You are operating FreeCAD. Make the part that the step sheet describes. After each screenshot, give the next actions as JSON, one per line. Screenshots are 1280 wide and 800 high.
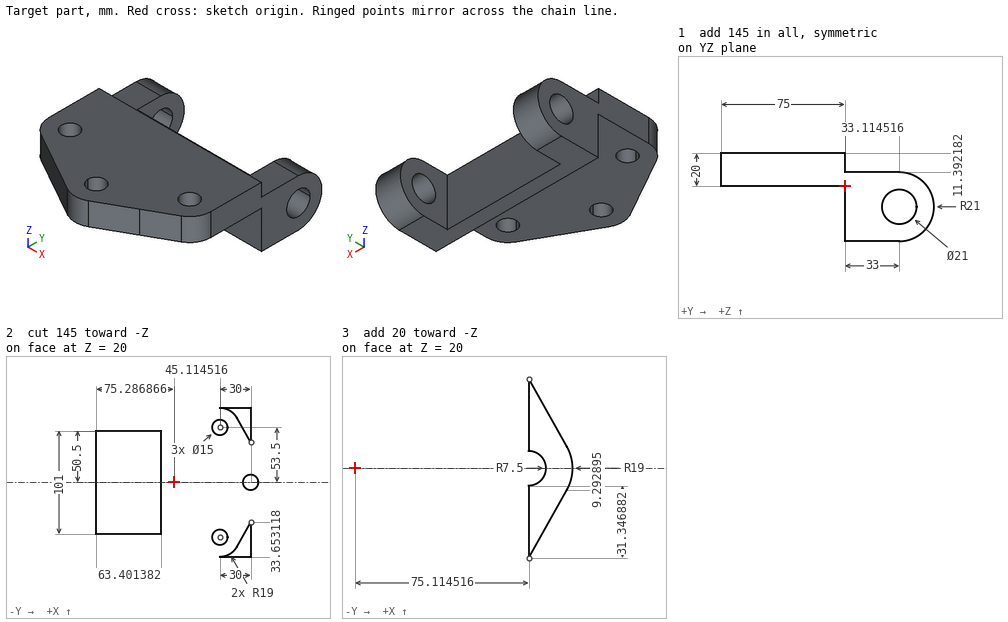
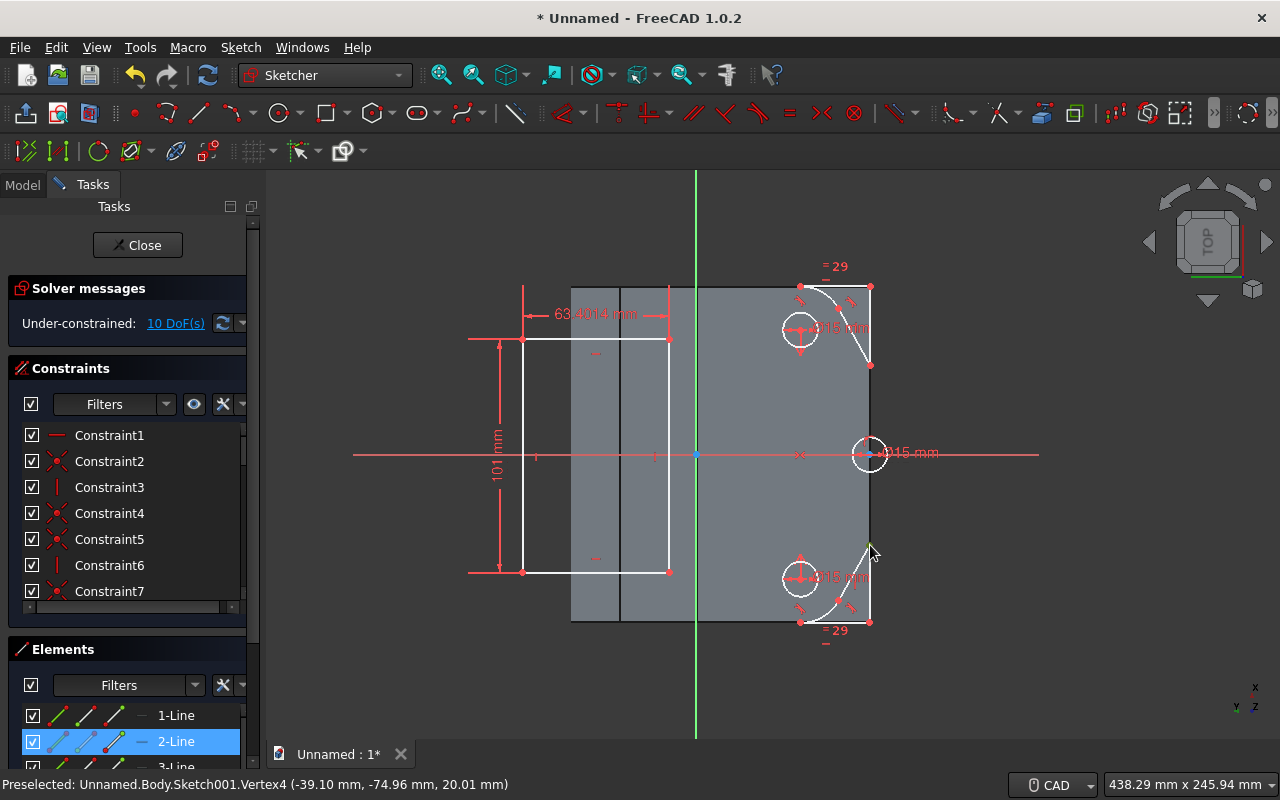
{"action": "left_click", "coordinate": [870, 366]}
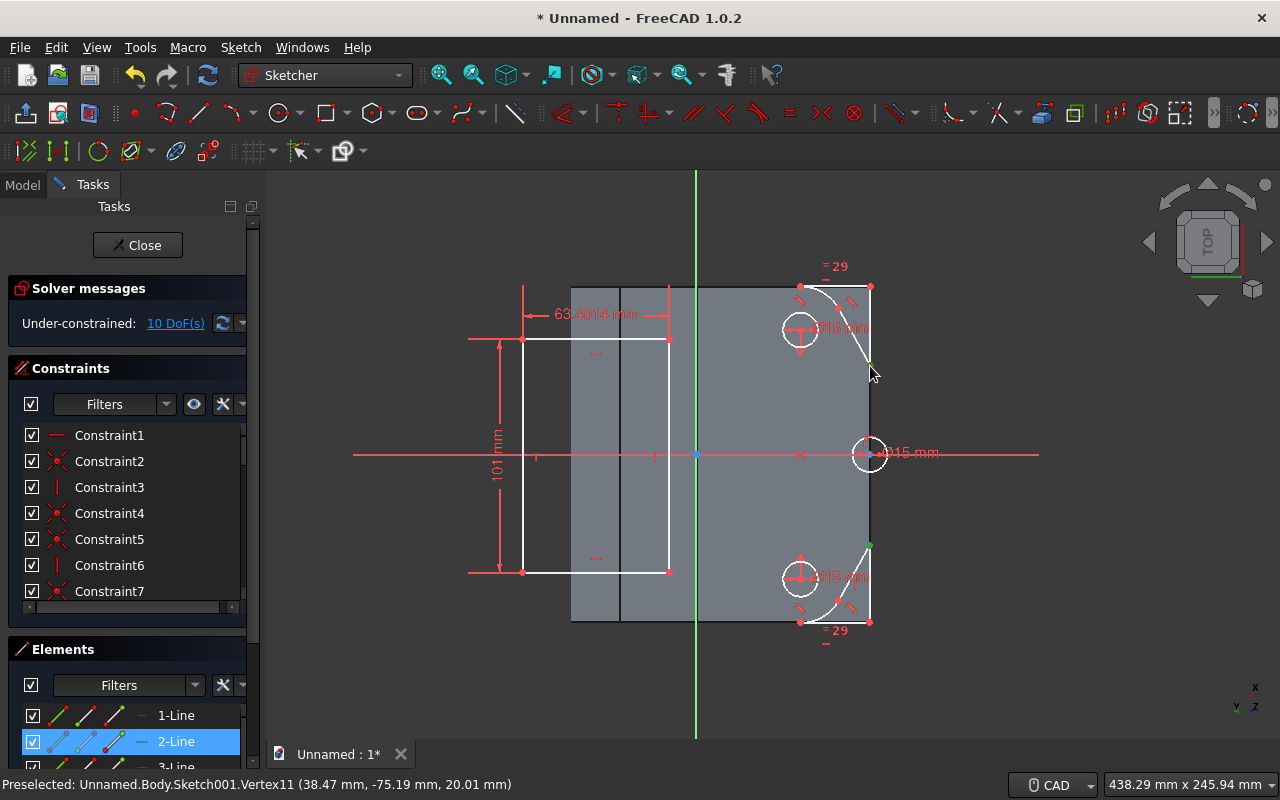
{"action": "left_click", "coordinate": [353, 455]}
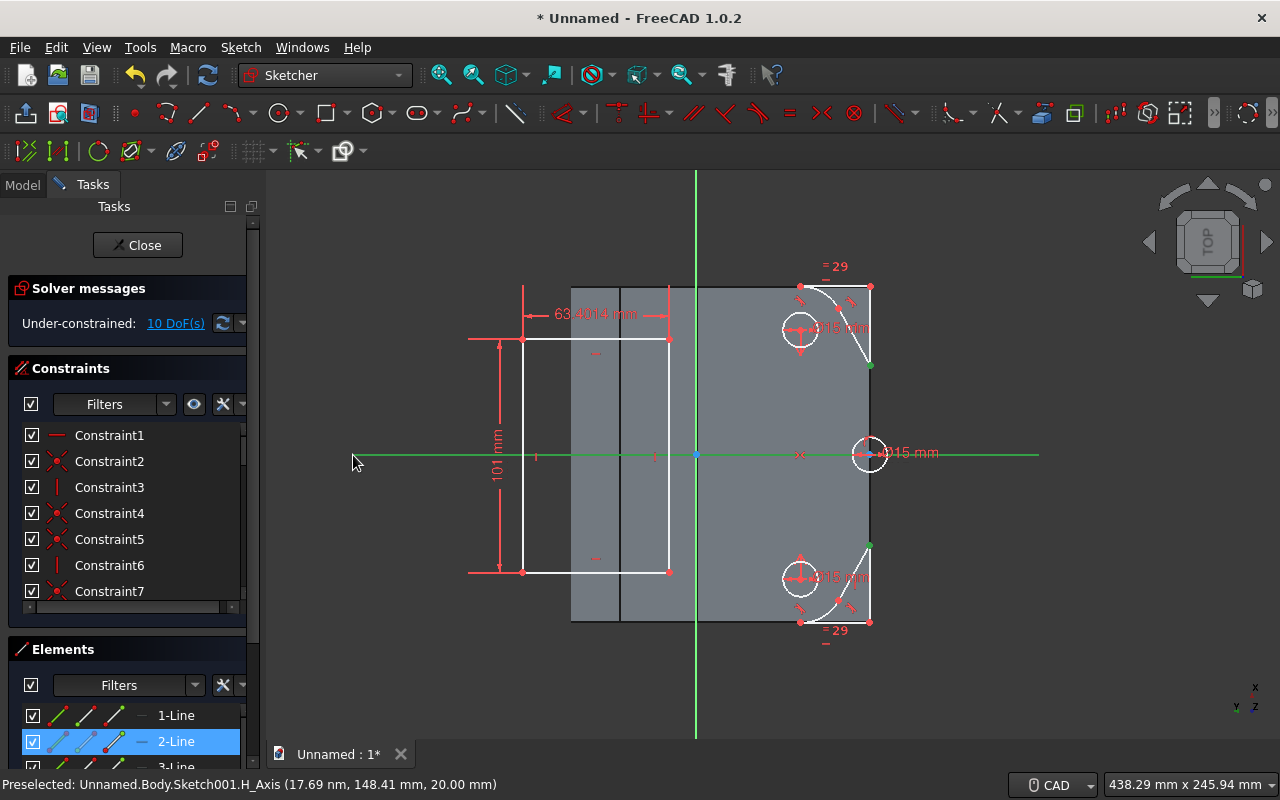
{"action": "left_click", "coordinate": [822, 114]}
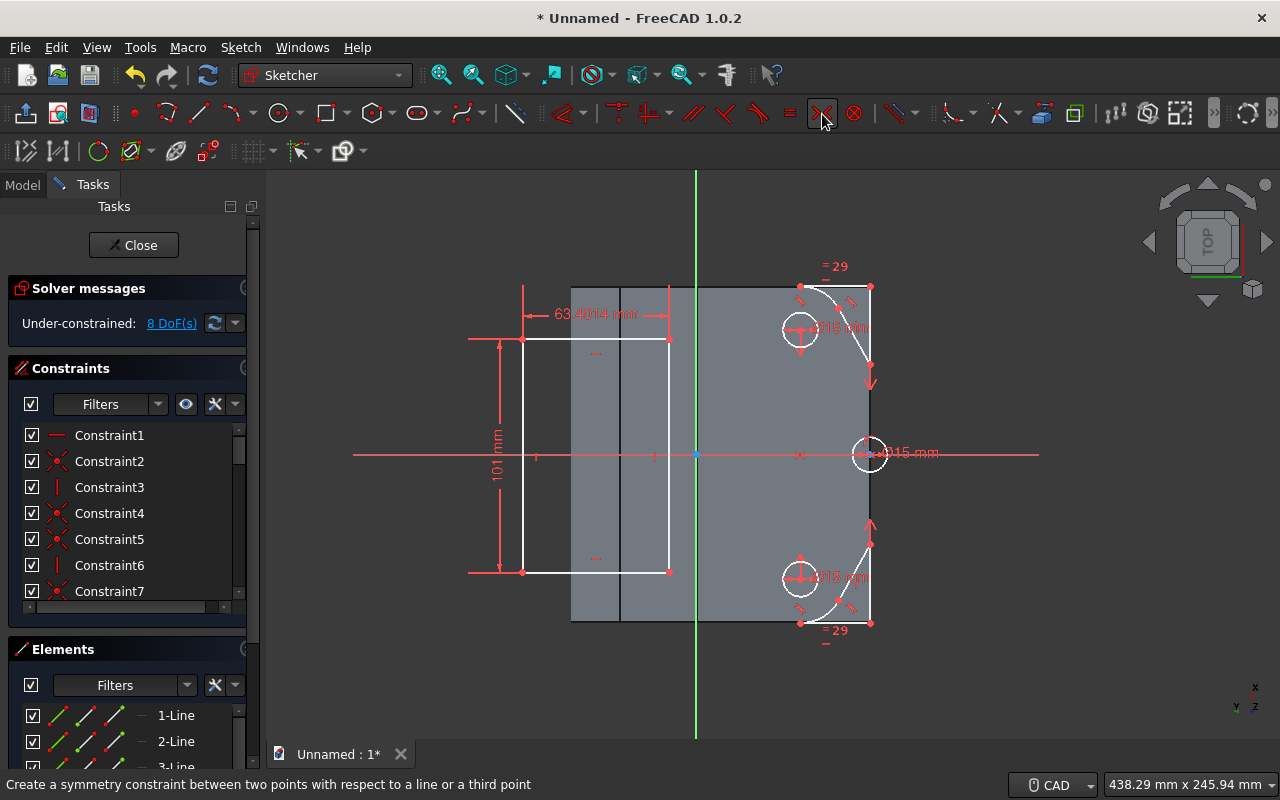
{"action": "left_click", "coordinate": [562, 114]}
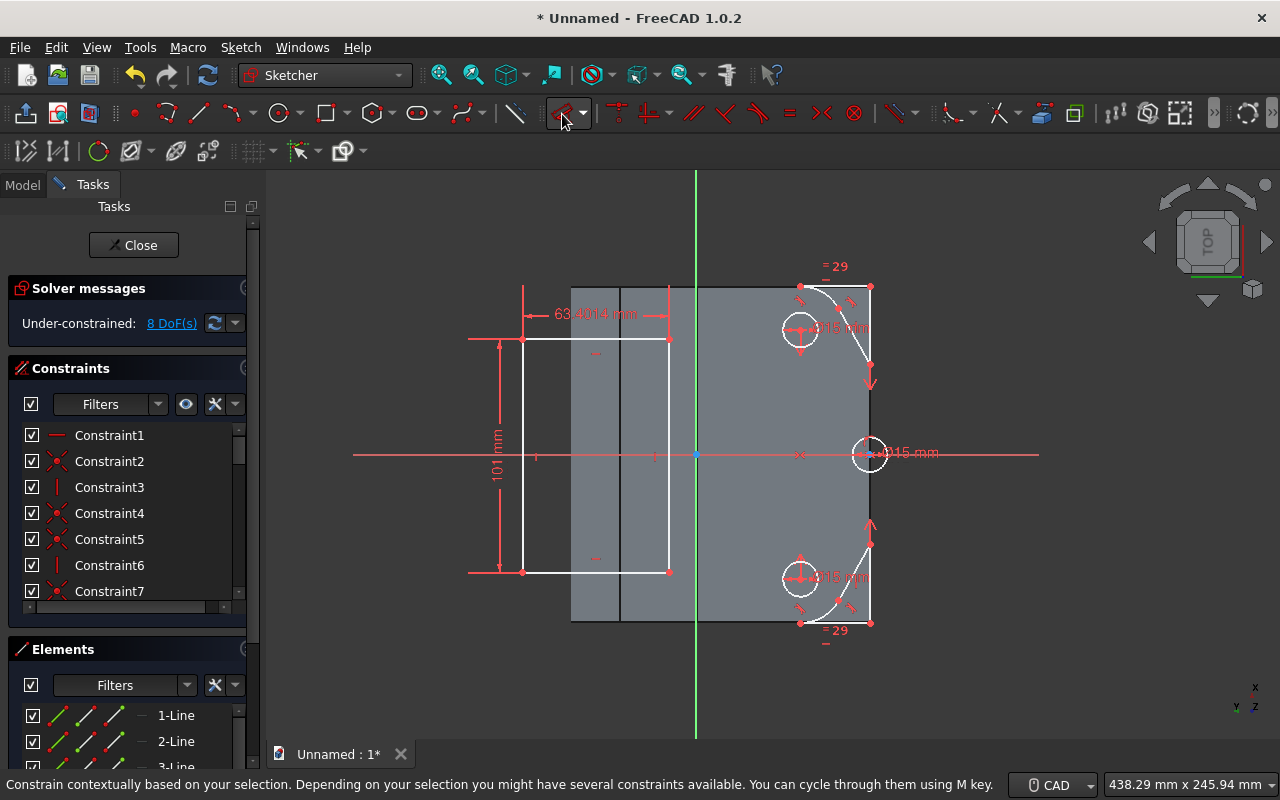
{"action": "left_click", "coordinate": [830, 612]}
{"action": "left_click", "coordinate": [818, 653]}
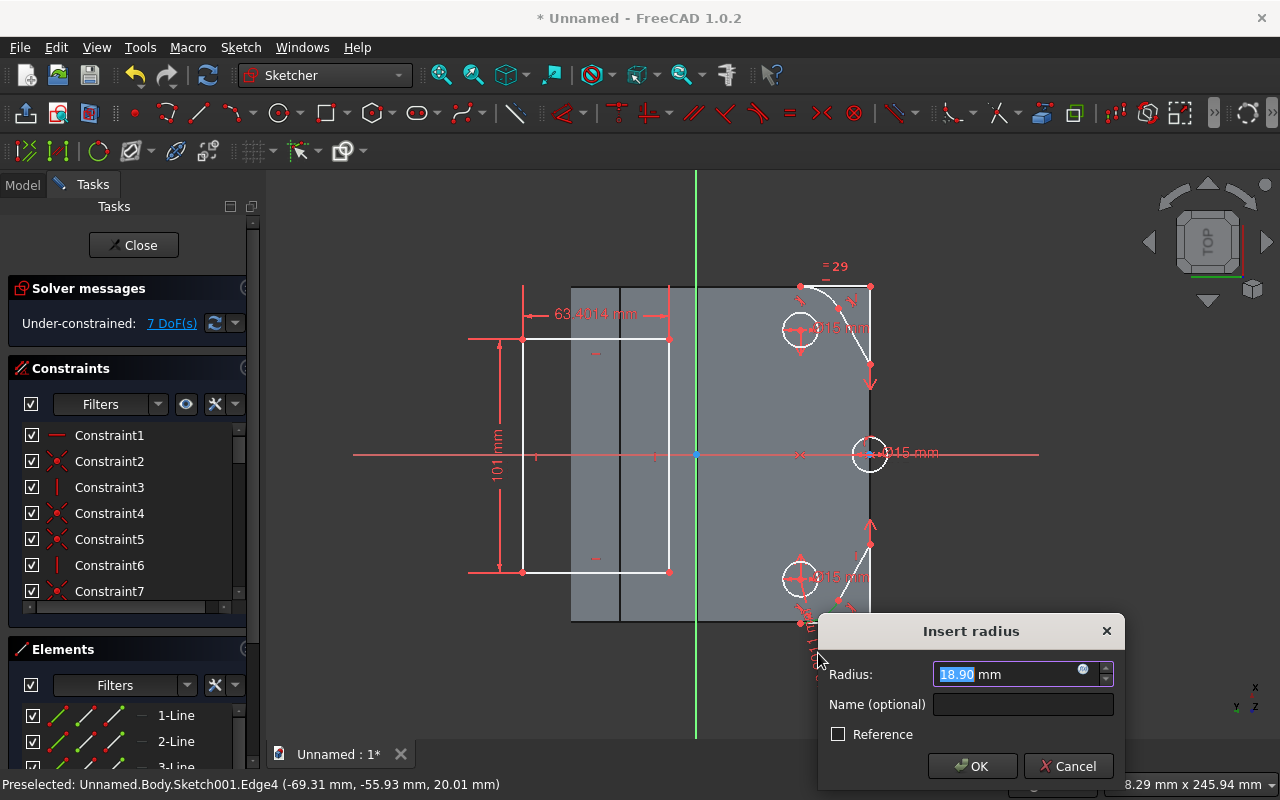
{"action": "type", "text": "19"}
{"action": "key", "text": "Return"}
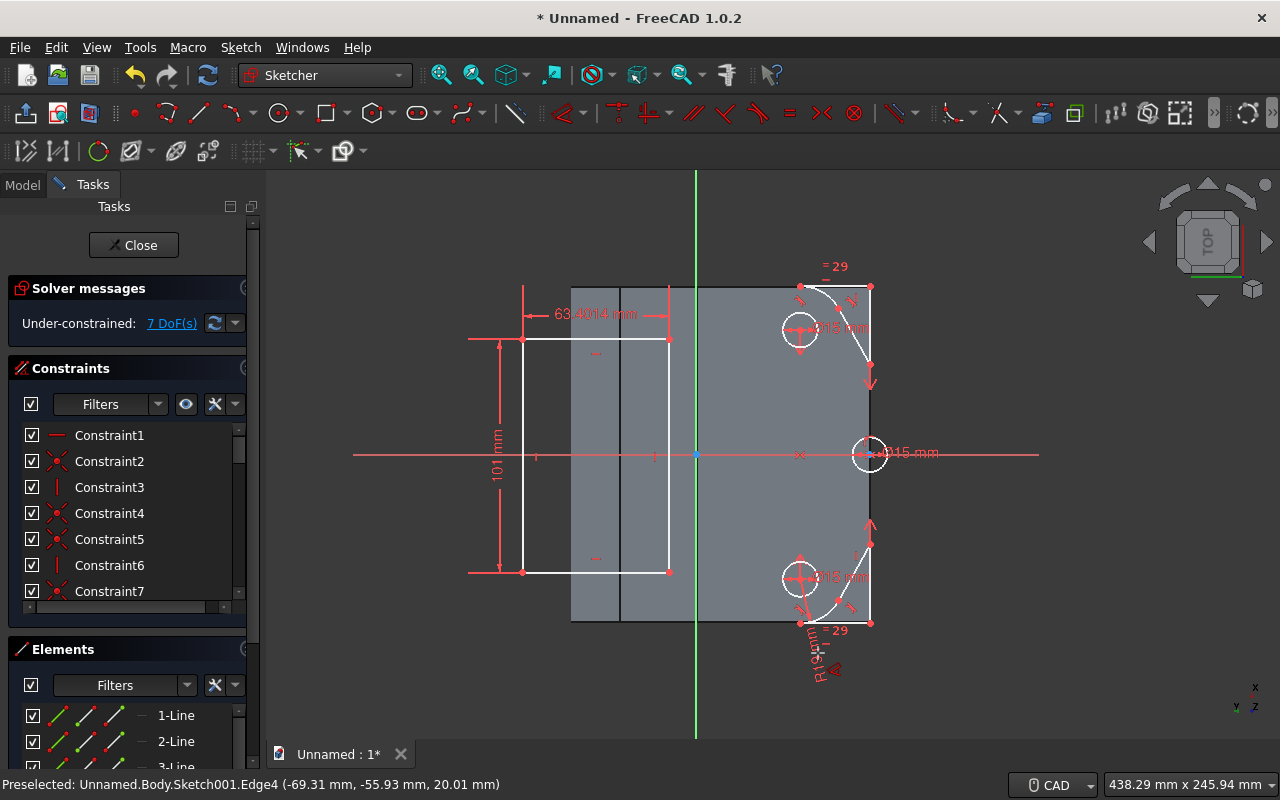
{"action": "left_click", "coordinate": [849, 623]}
{"action": "left_click", "coordinate": [835, 681]}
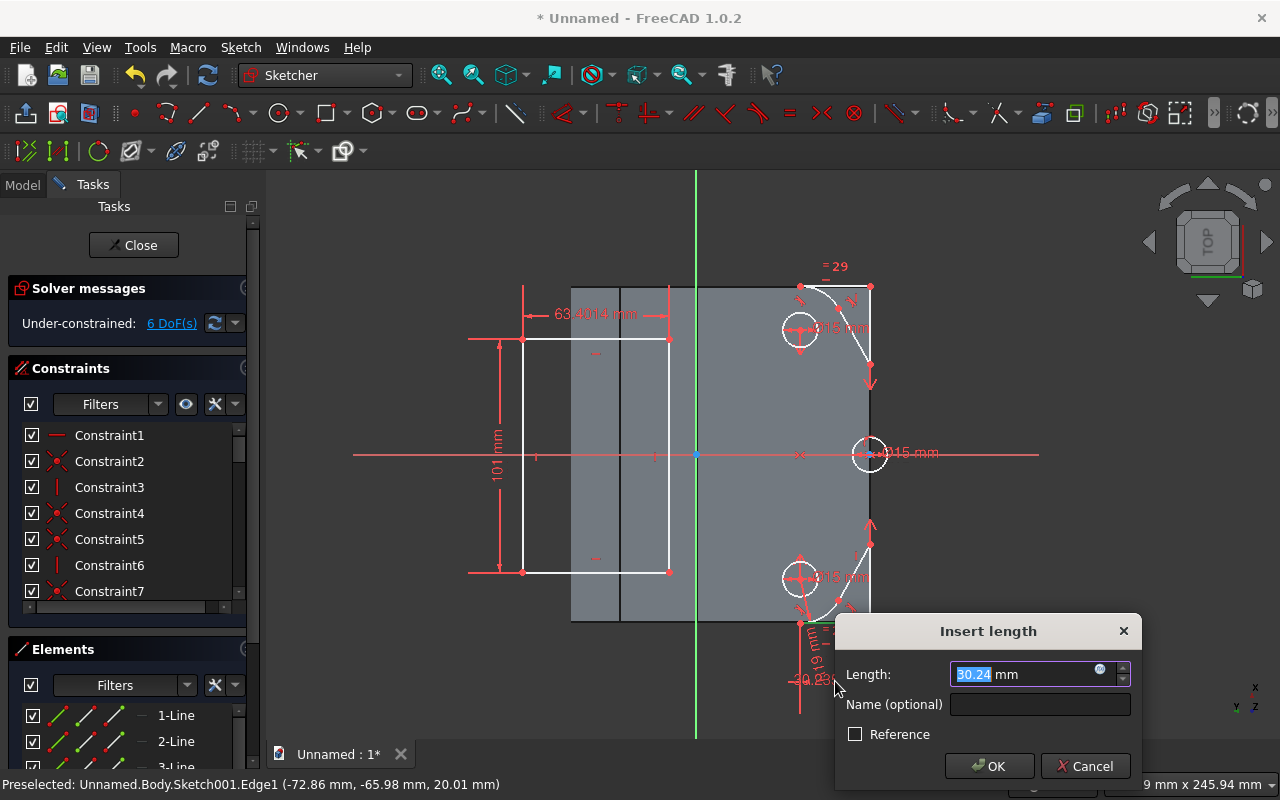
{"action": "type", "text": "30"}
{"action": "key", "text": "Return"}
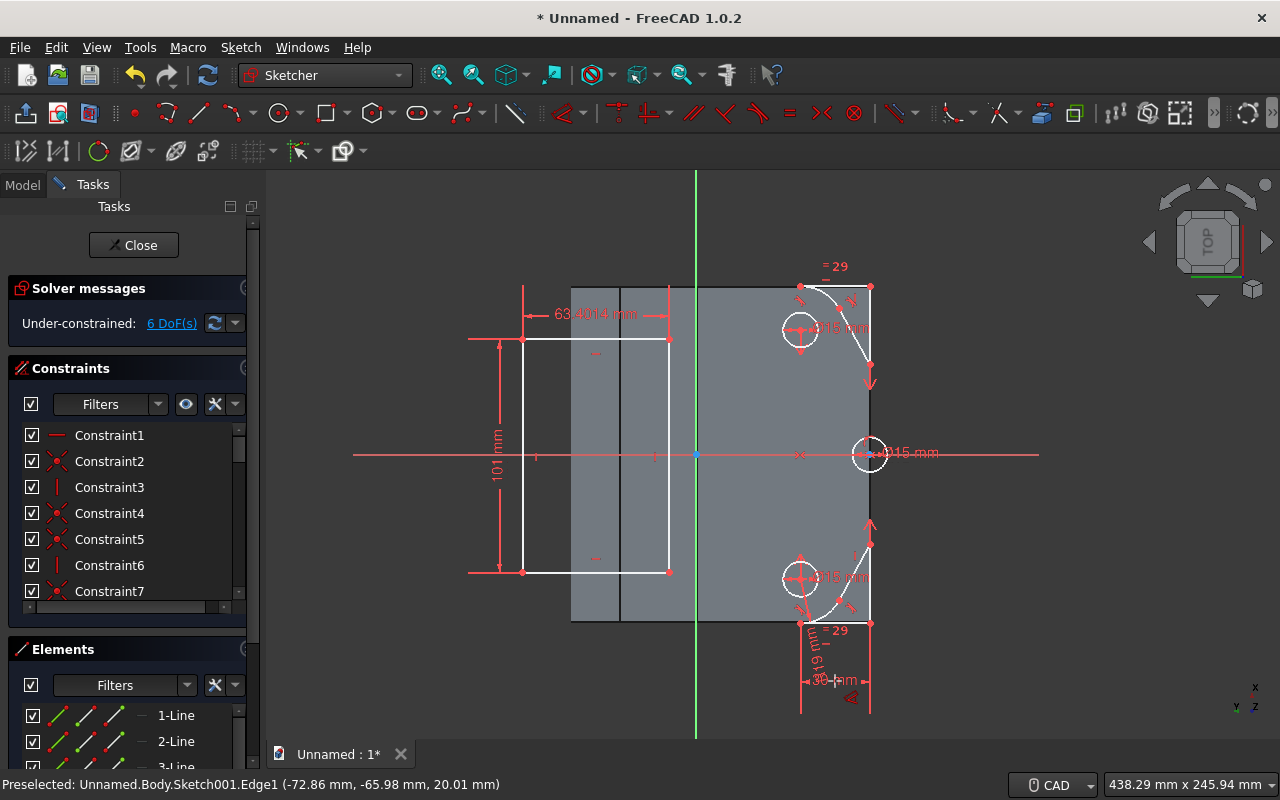
{"action": "left_click", "coordinate": [801, 330]}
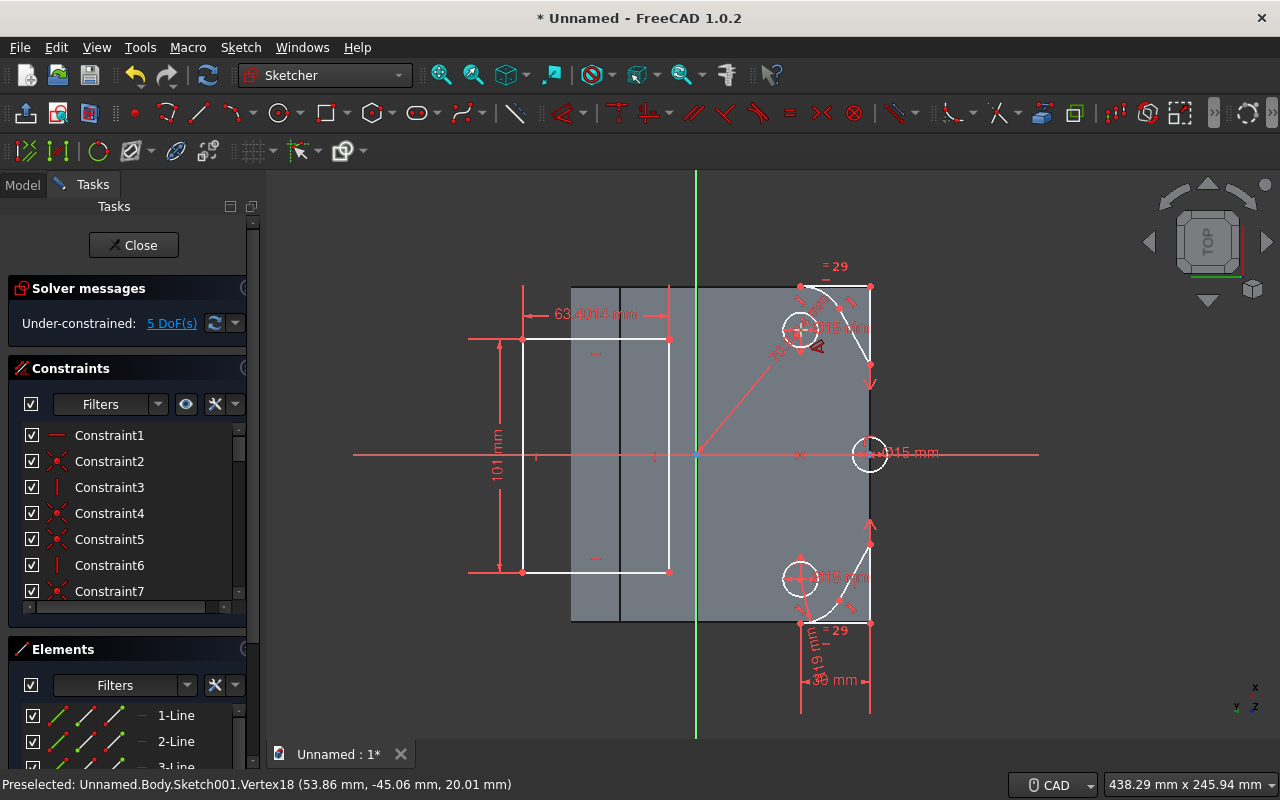
{"action": "left_click", "coordinate": [870, 455]}
{"action": "left_click", "coordinate": [835, 489]}